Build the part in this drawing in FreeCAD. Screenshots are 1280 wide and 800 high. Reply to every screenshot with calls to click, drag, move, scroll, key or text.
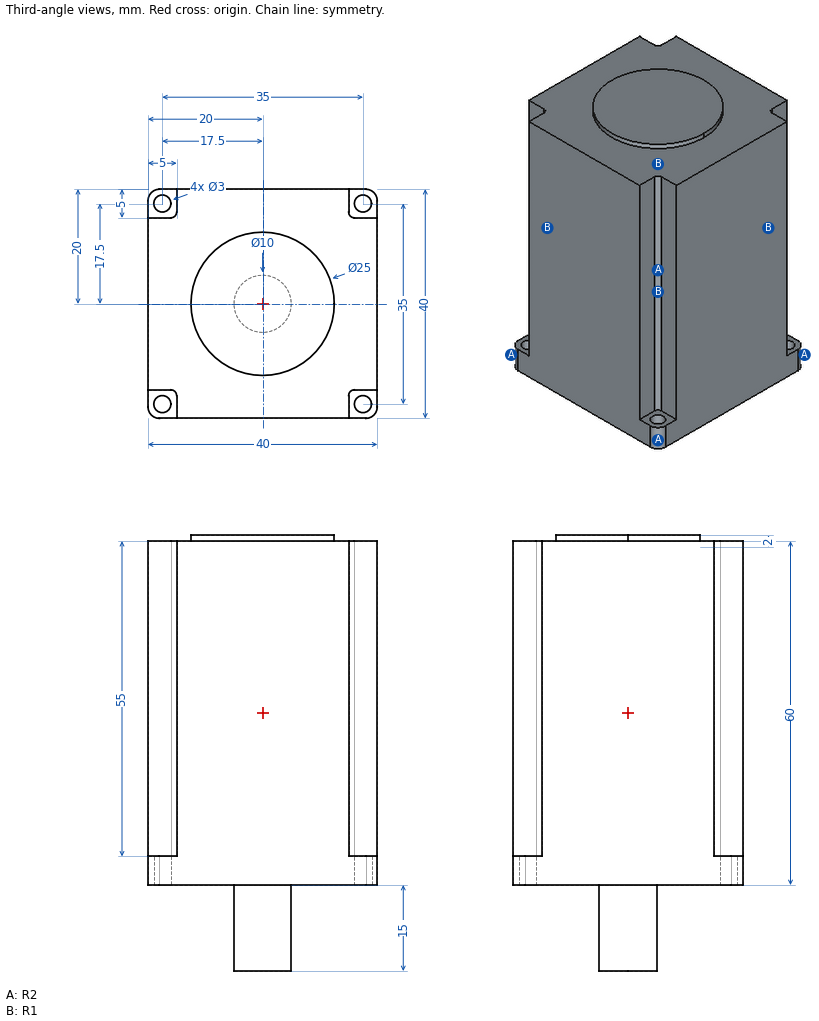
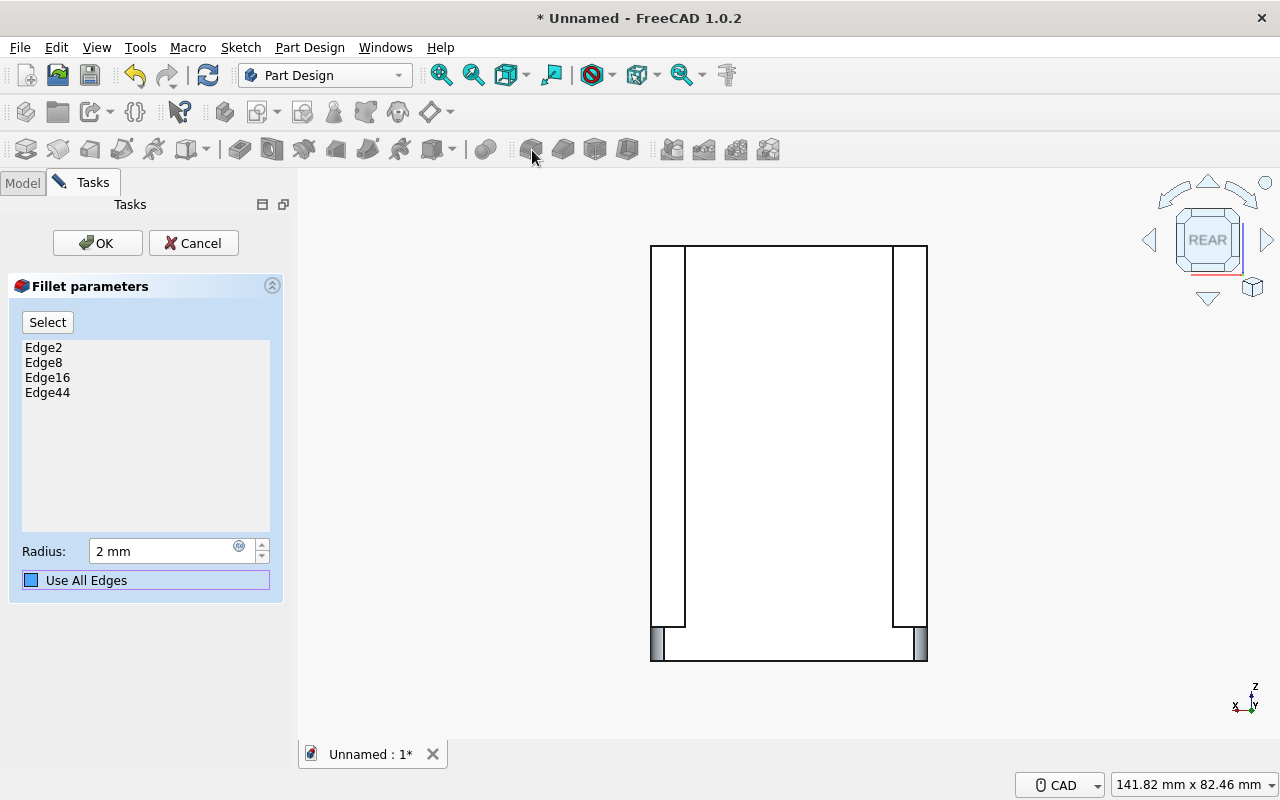
click(98, 243)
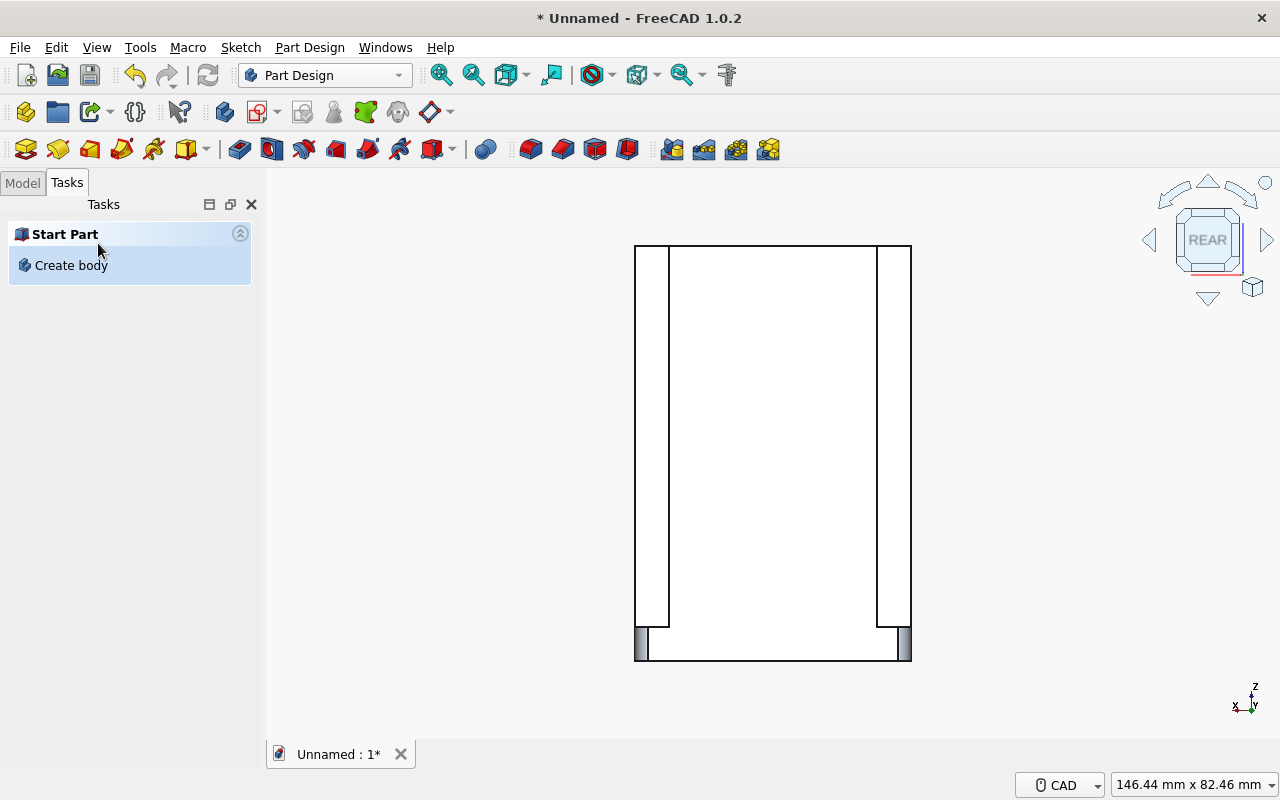
key(0)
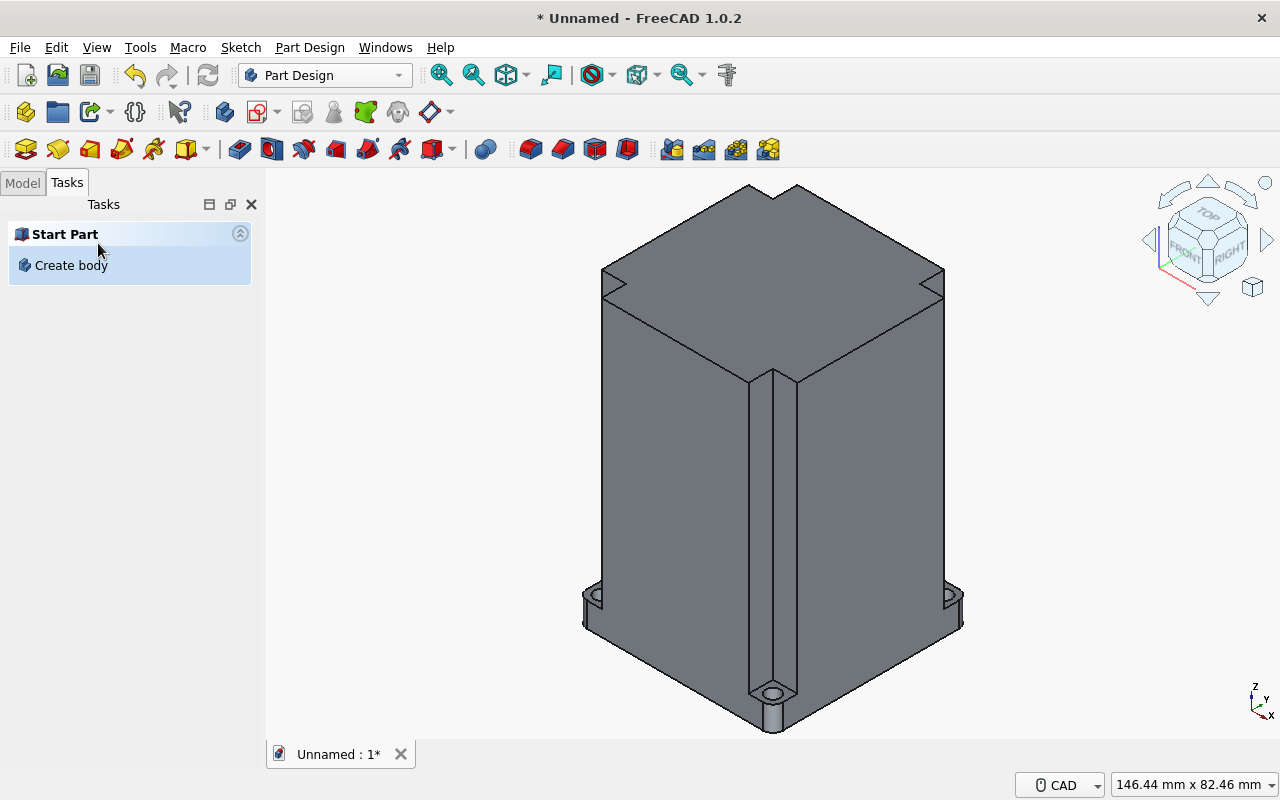
click(773, 283)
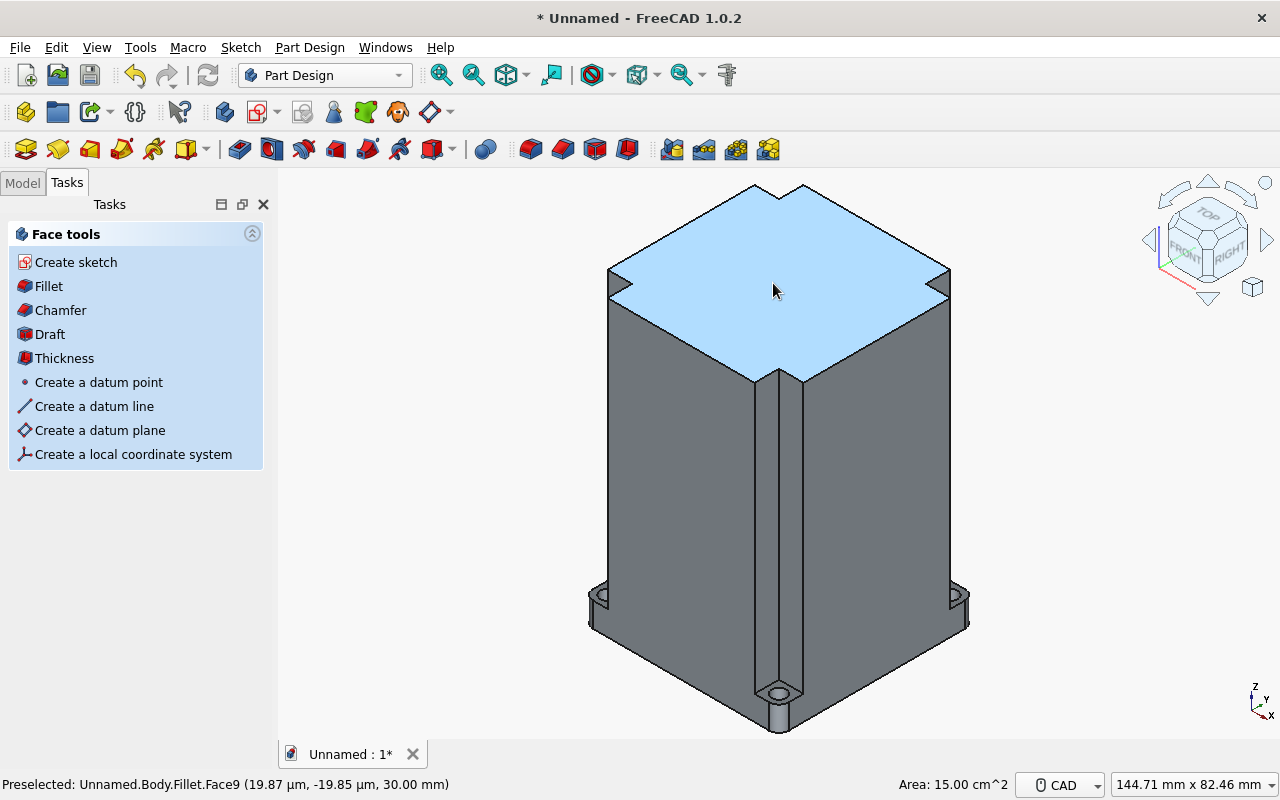
click(258, 112)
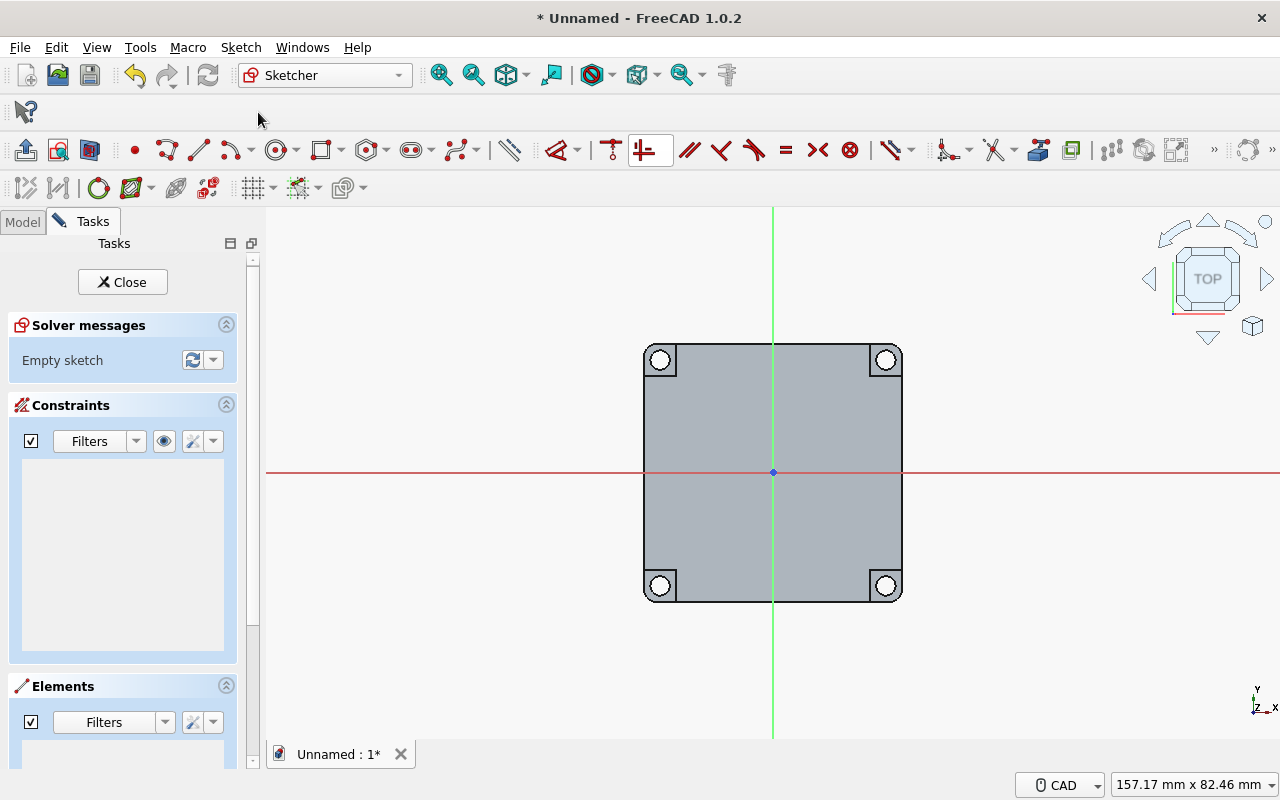
scroll(829, 473, up, 4)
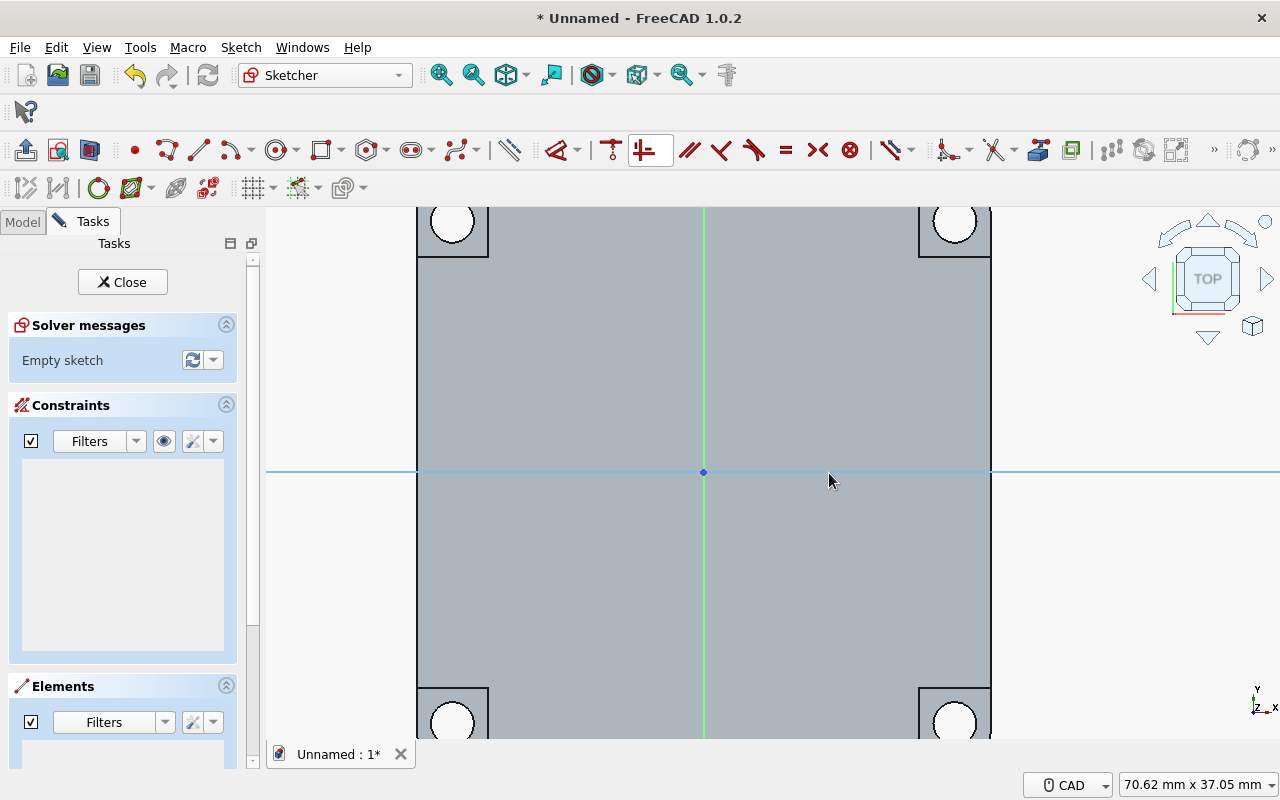
click(276, 150)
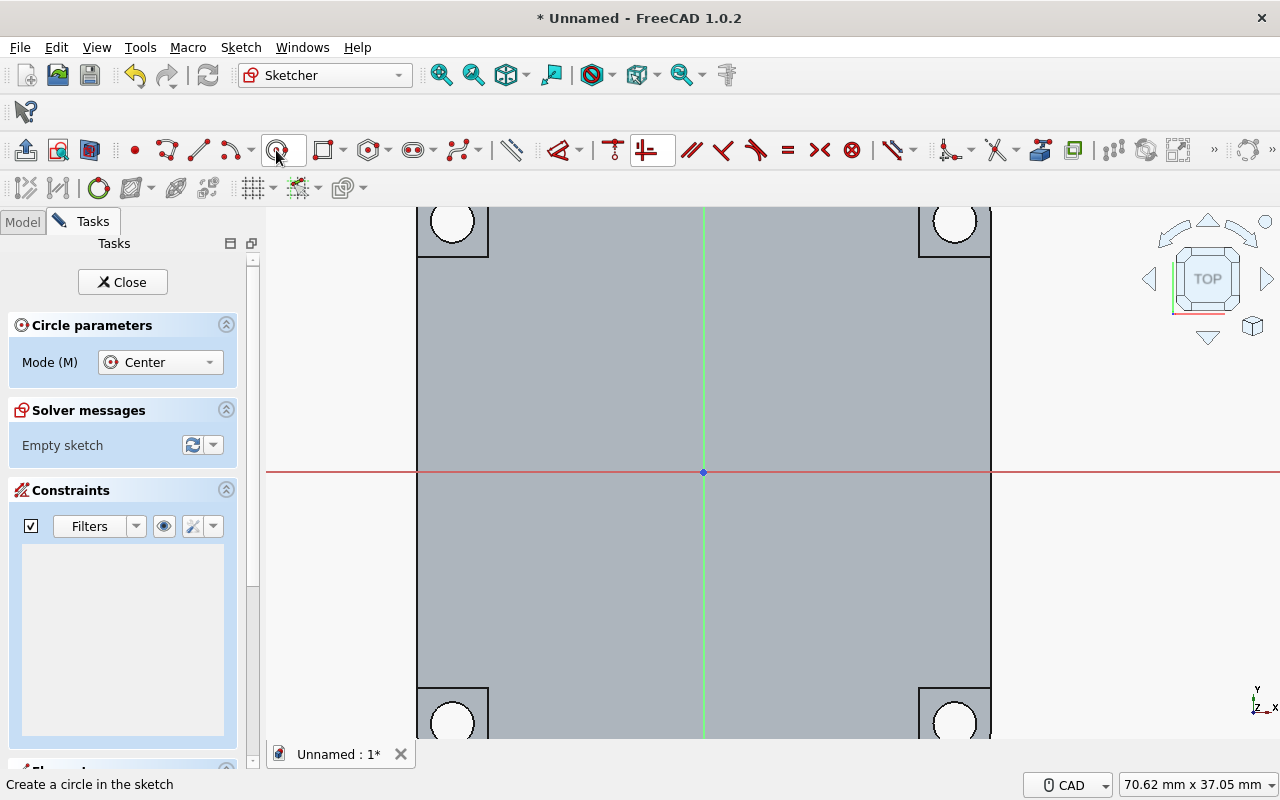
click(704, 472)
click(831, 345)
key(Escape)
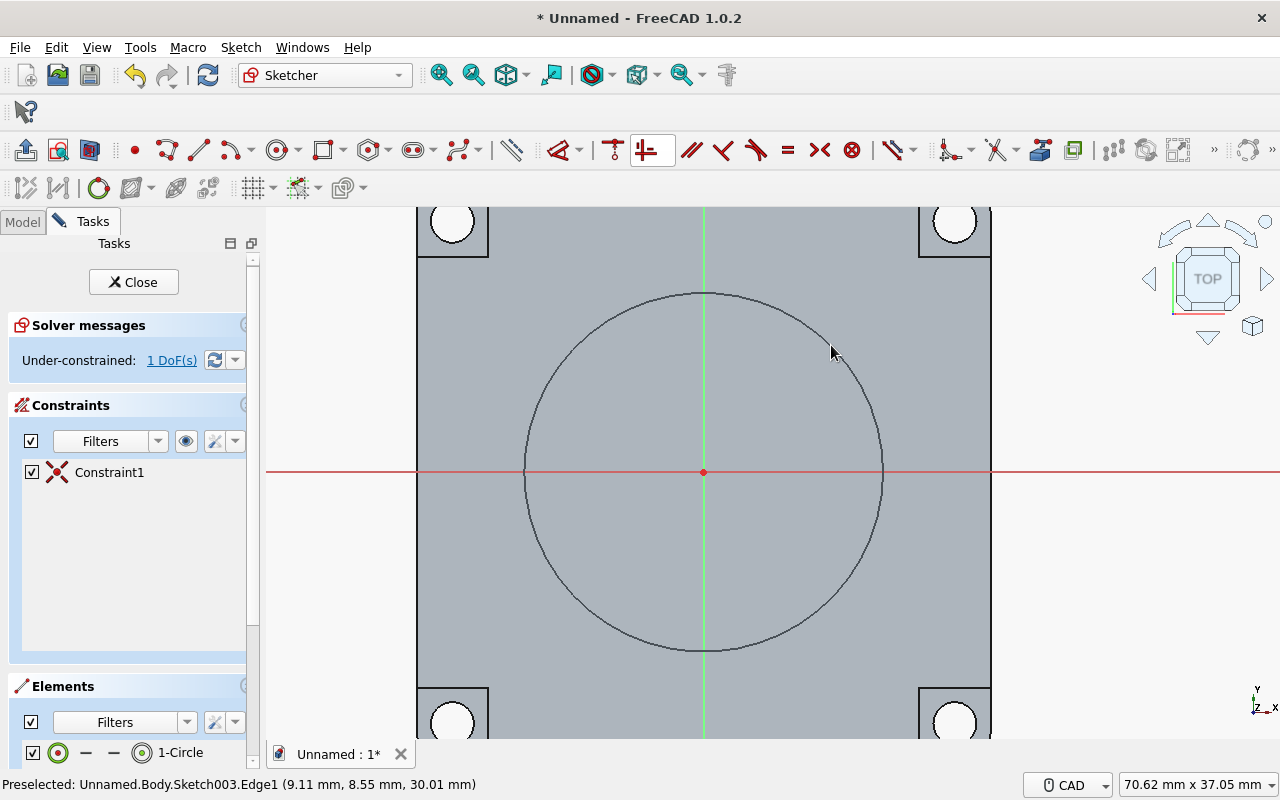
click(558, 150)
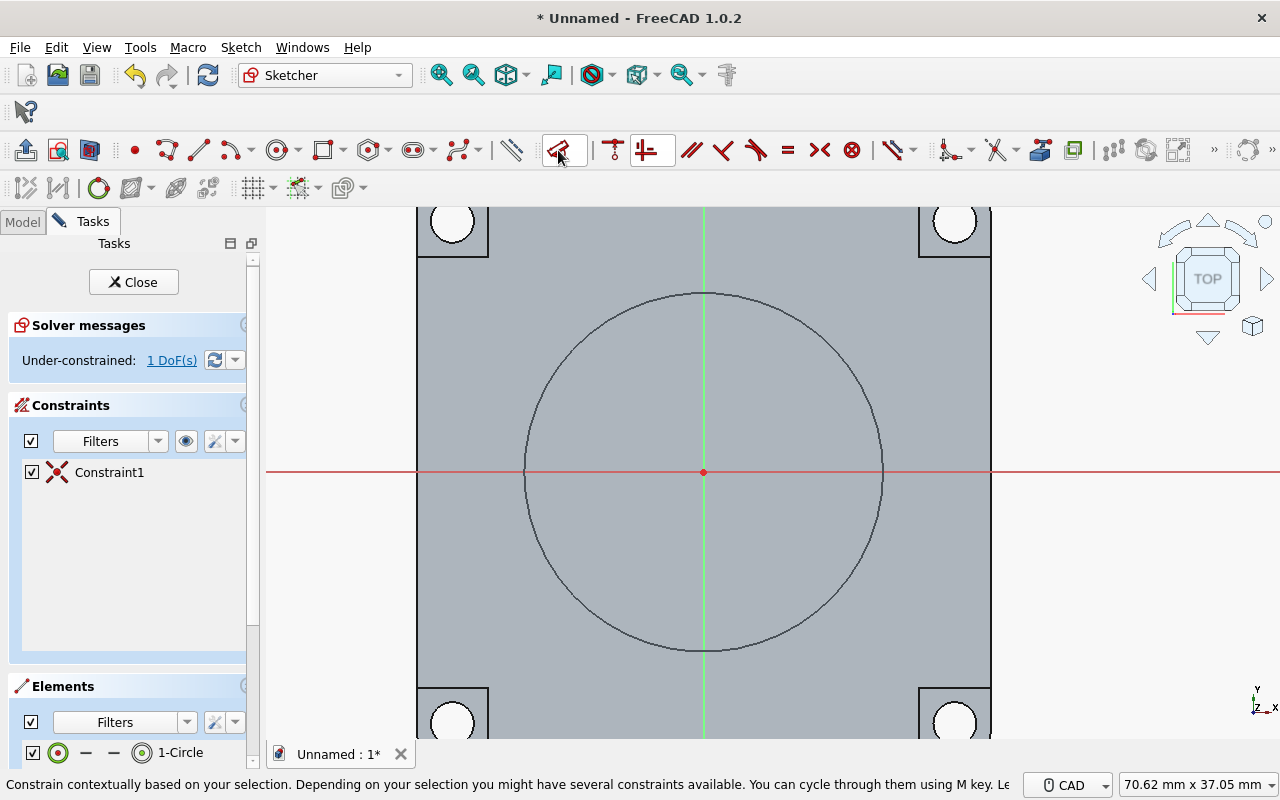
click(830, 345)
click(853, 322)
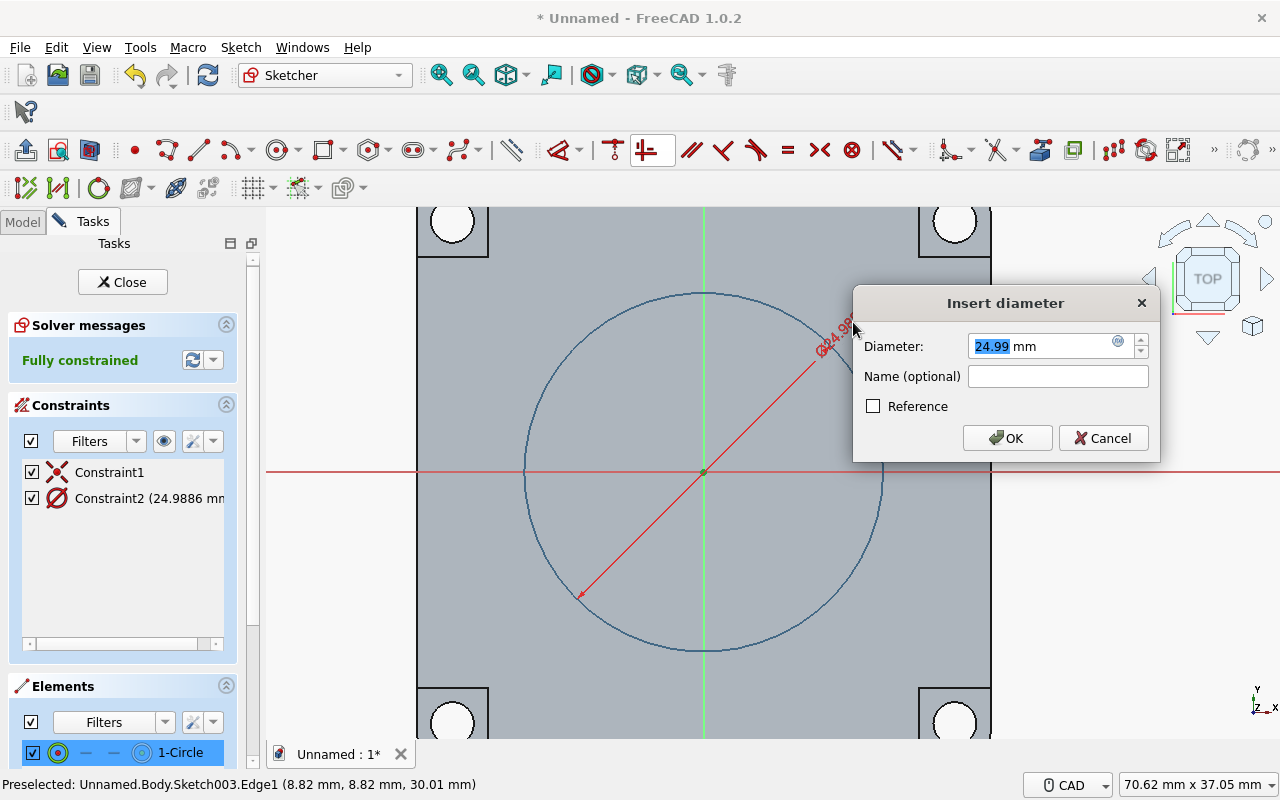
text(25)
key(Return)
key(Escape)